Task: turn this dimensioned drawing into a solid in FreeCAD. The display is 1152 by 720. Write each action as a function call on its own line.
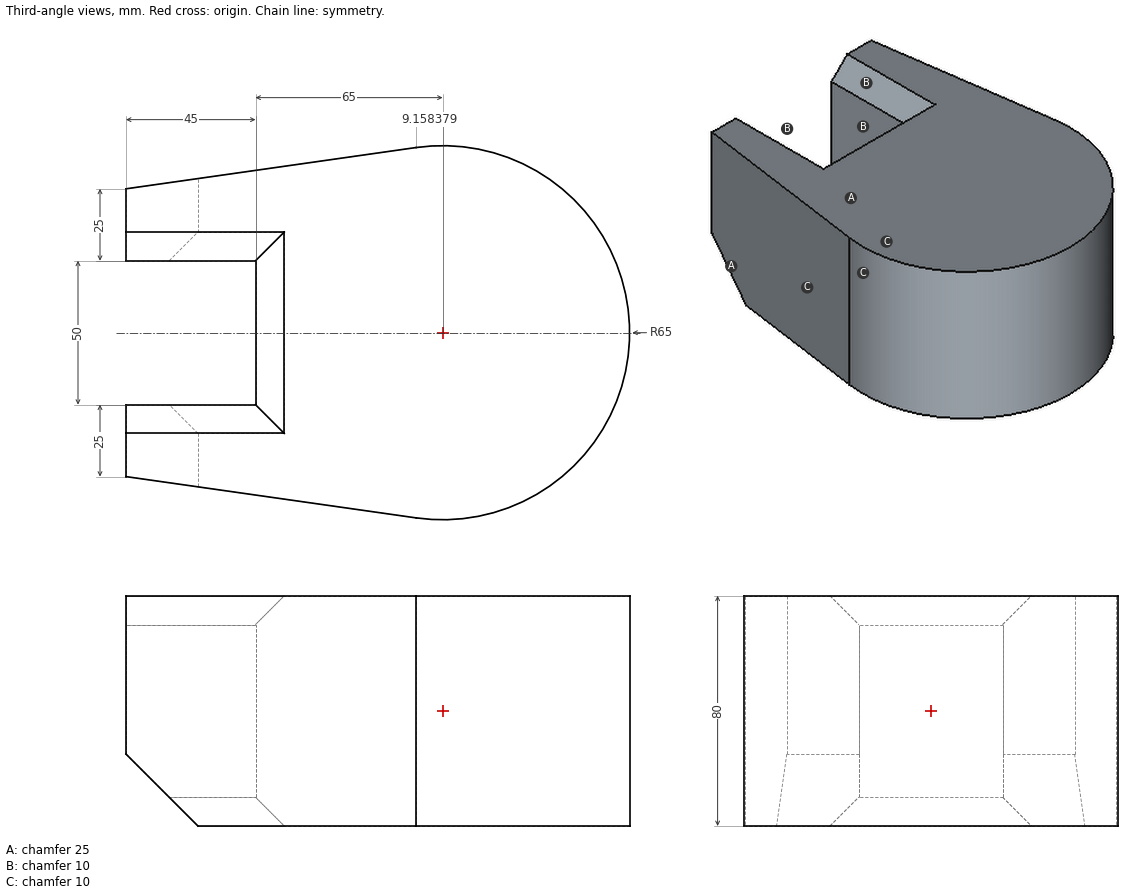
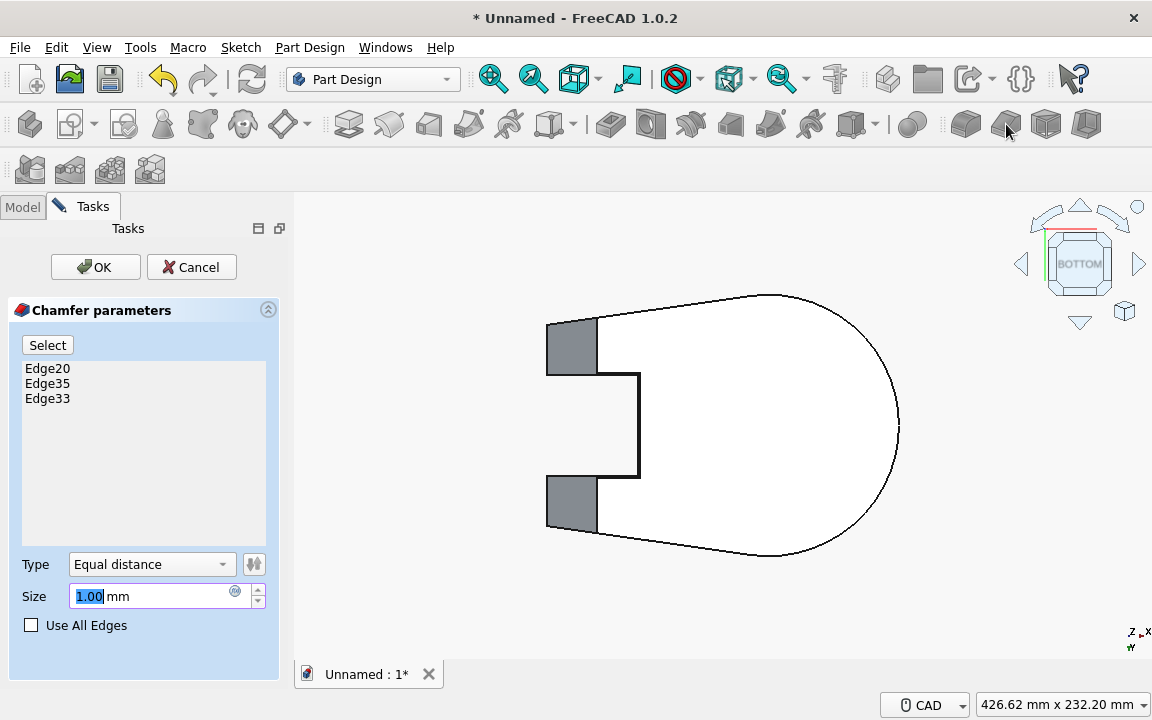
text(10)
key(Tab)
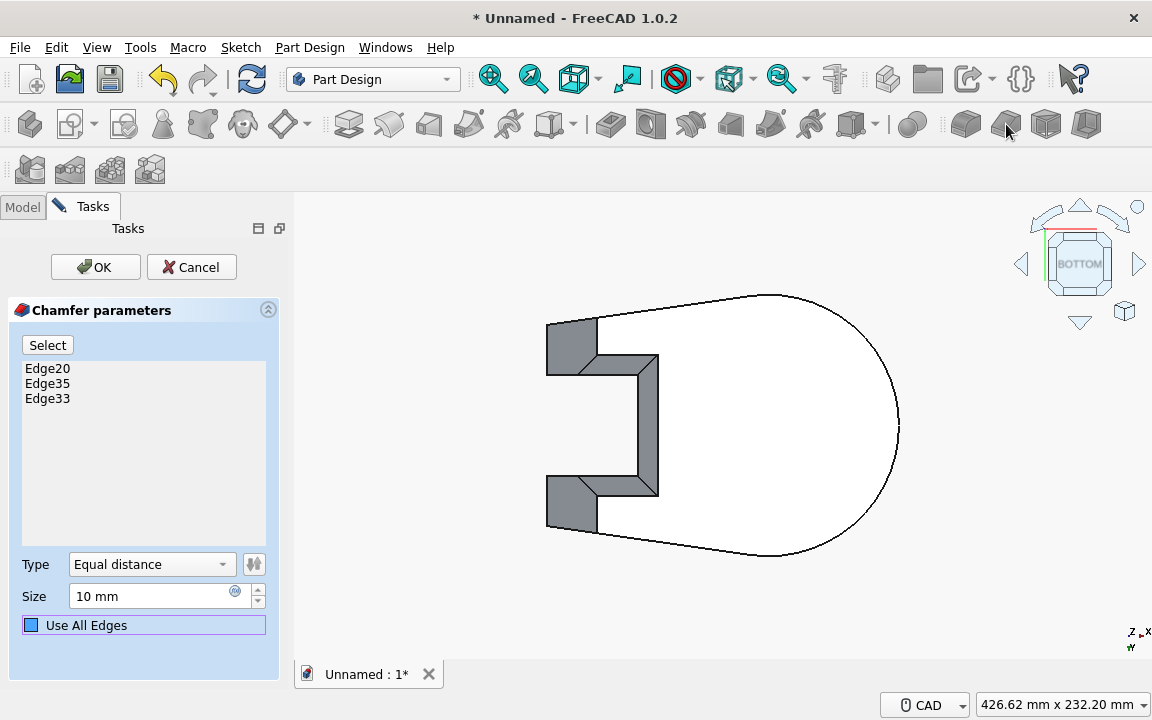
click(96, 267)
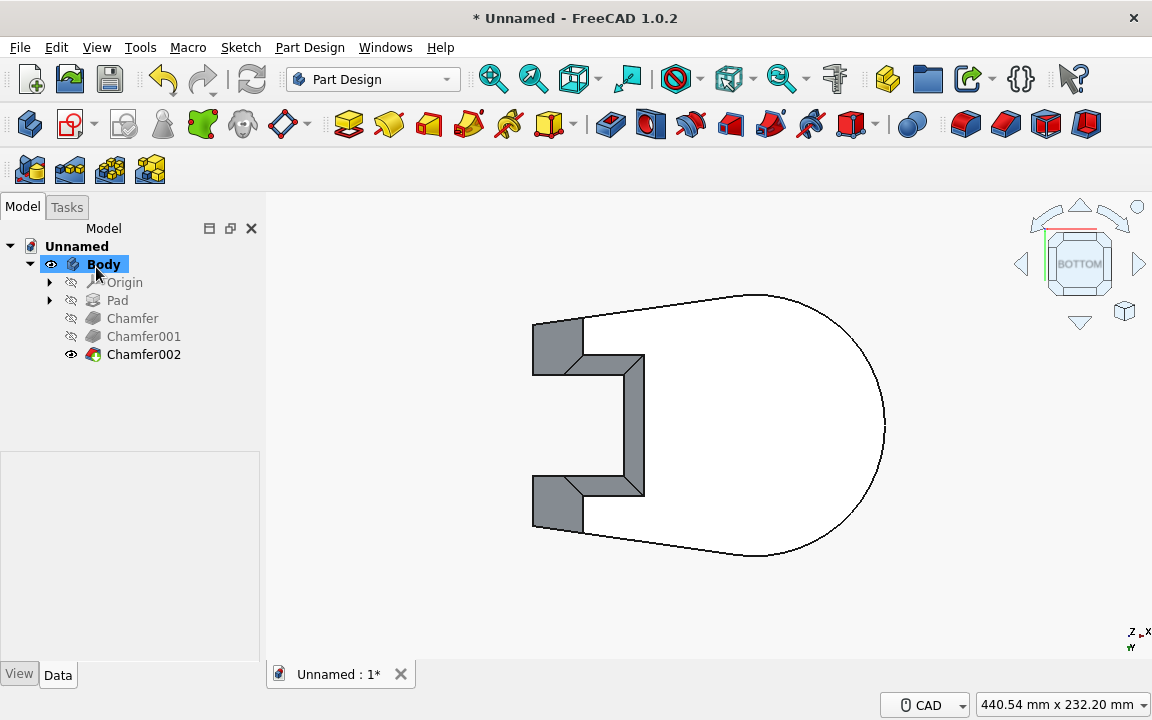
key(0)